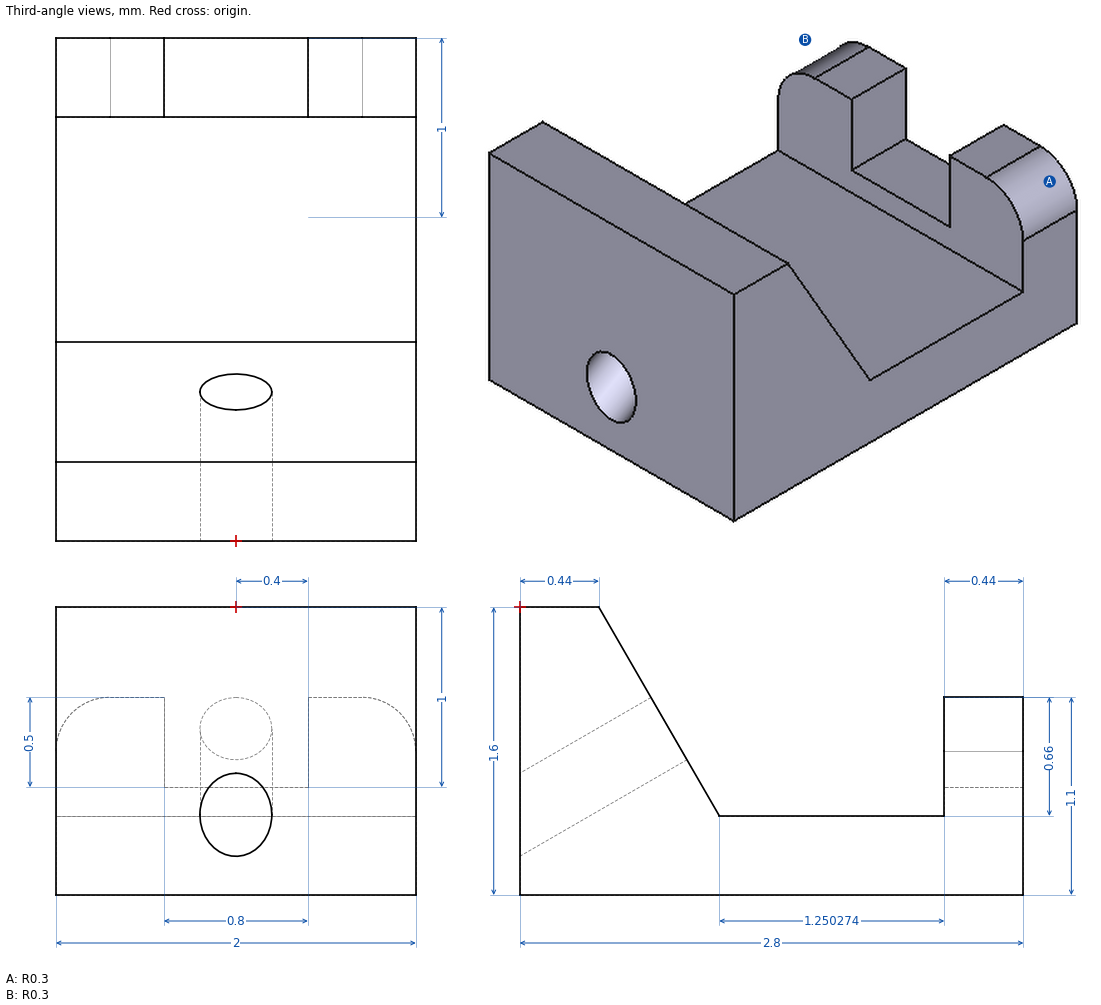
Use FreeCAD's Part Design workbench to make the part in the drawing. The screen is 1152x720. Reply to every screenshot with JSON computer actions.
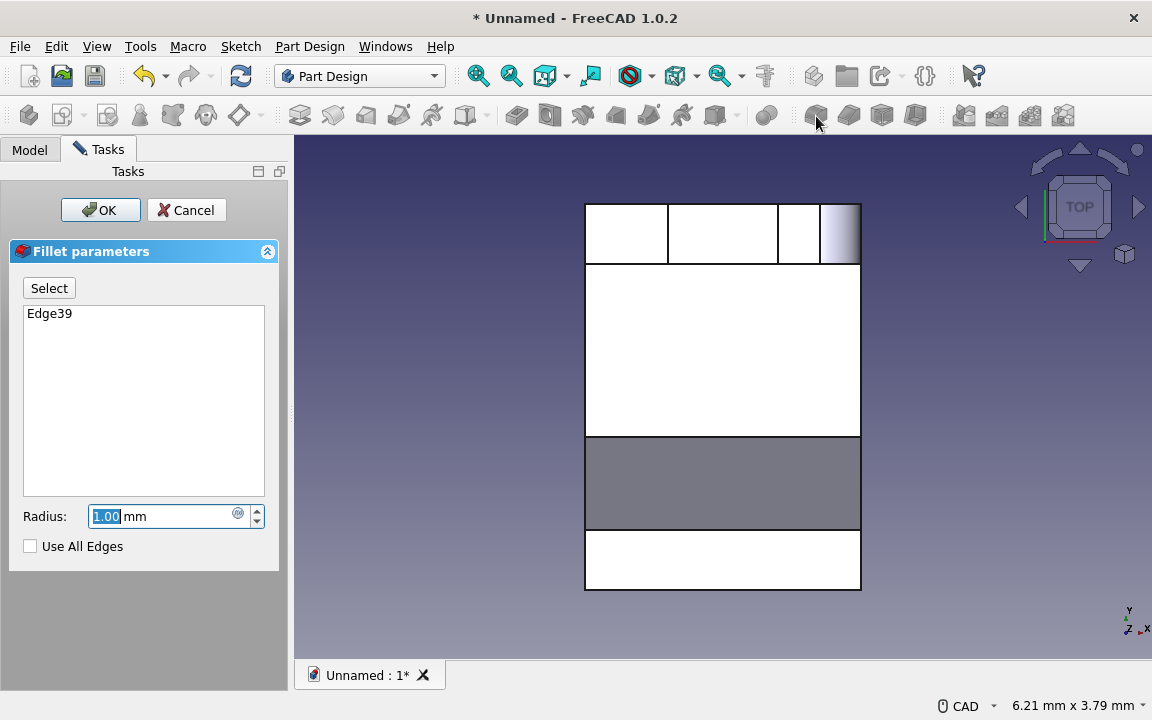
{"action": "type", "text": "0.3"}
{"action": "key", "text": "Tab"}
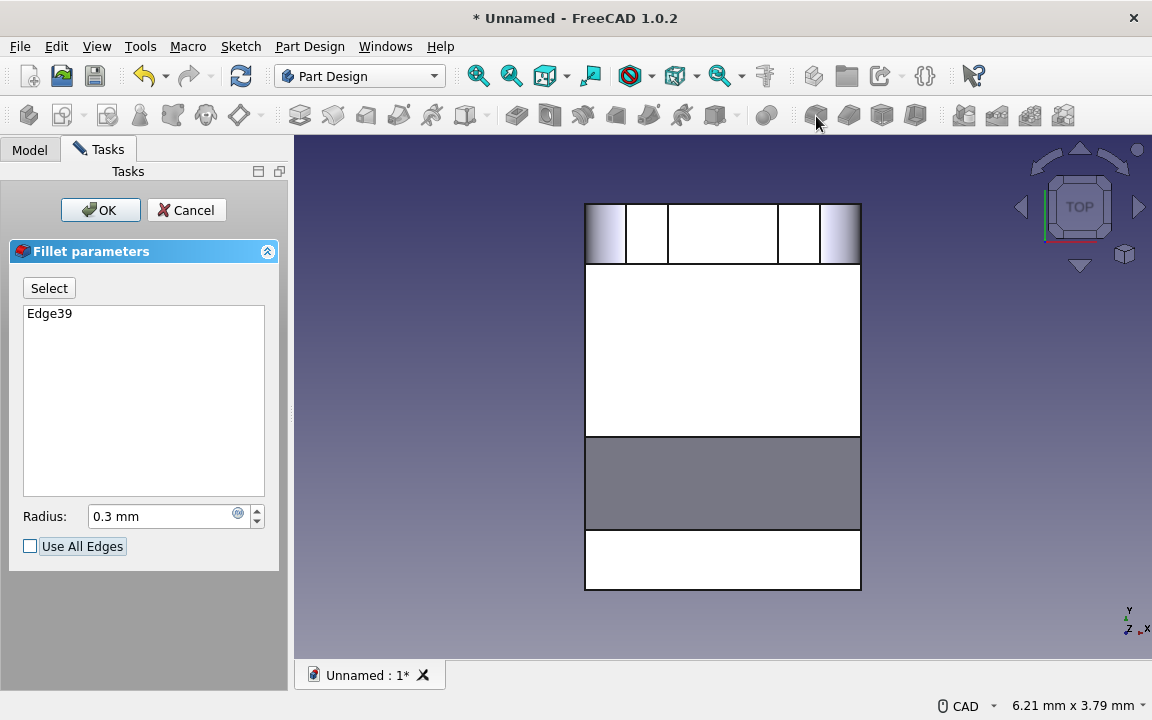
{"action": "left_click", "coordinate": [101, 210]}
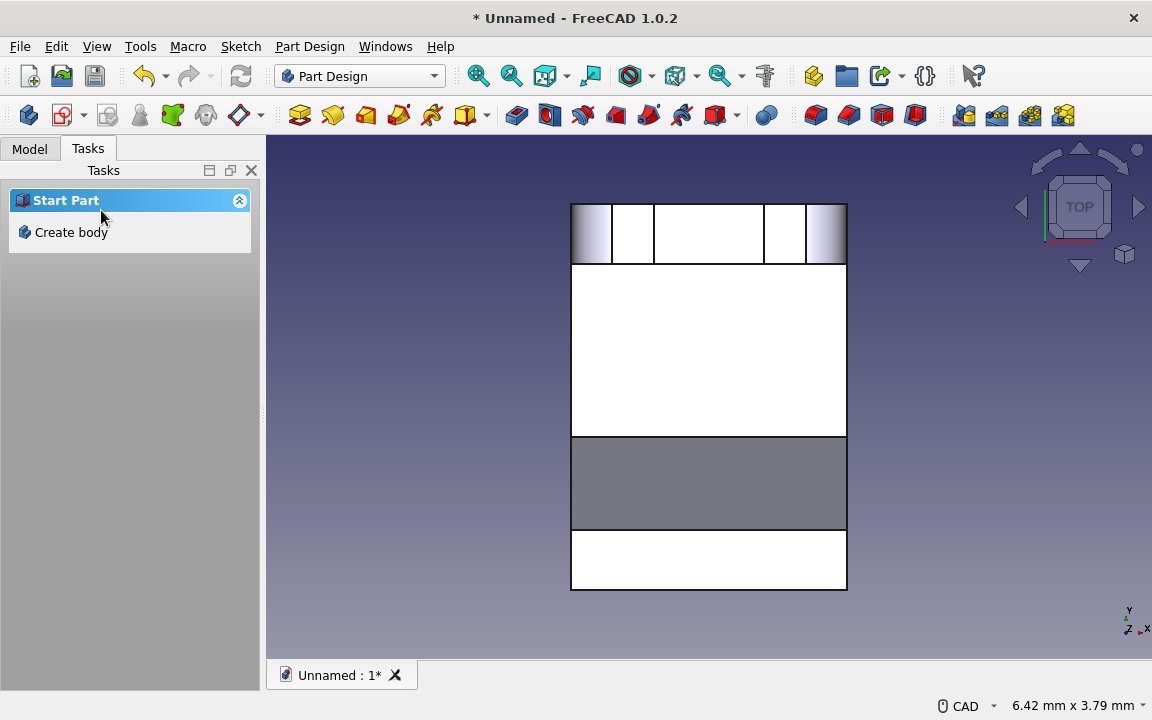
{"action": "left_click", "coordinate": [670, 482]}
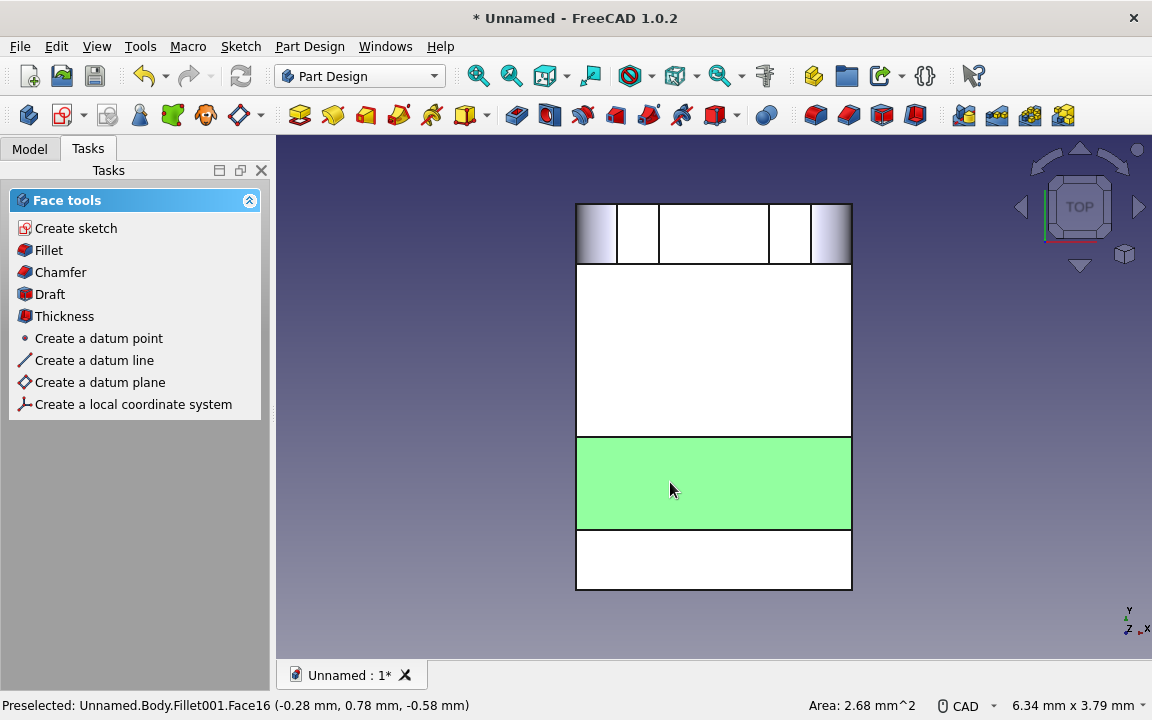
{"action": "left_click", "coordinate": [62, 116]}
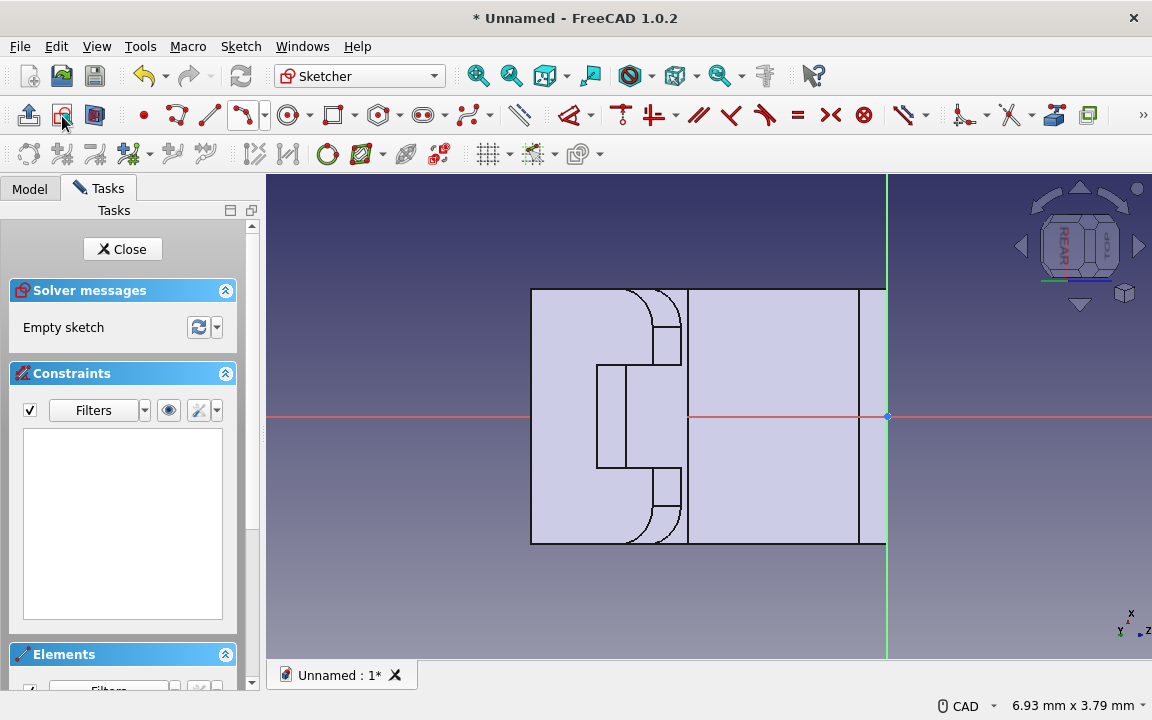
{"action": "scroll", "coordinate": [783, 416], "scroll_direction": "up", "scroll_amount": 9}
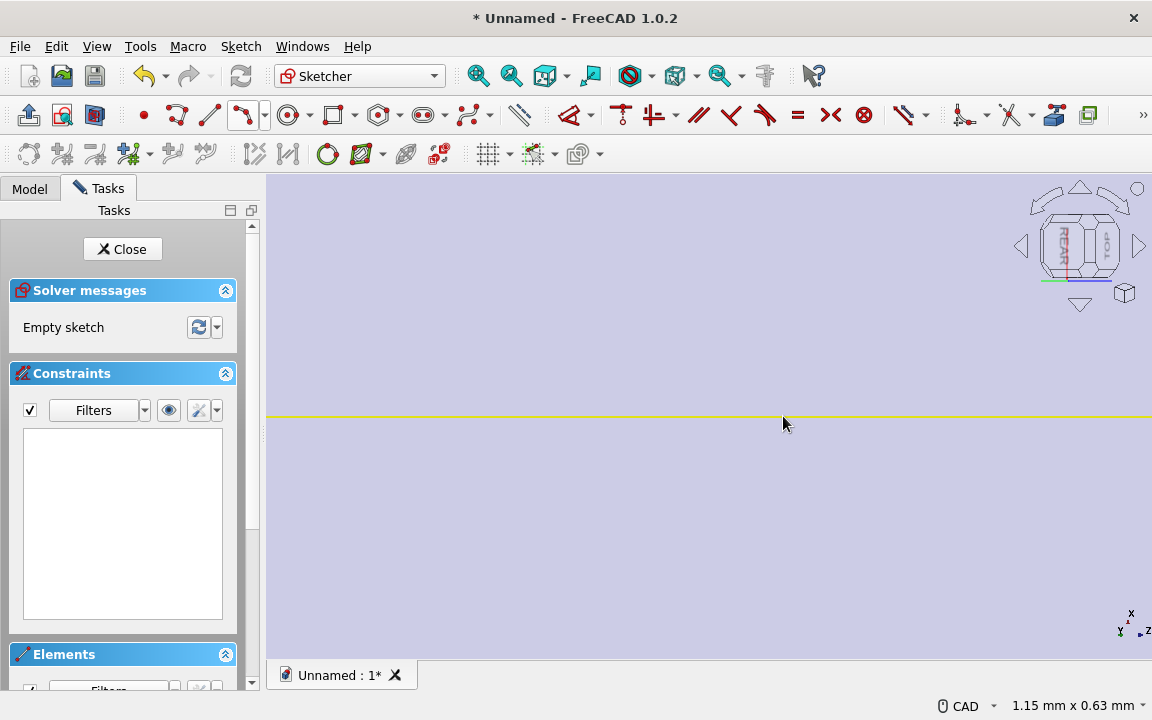
{"action": "key", "text": "g c"}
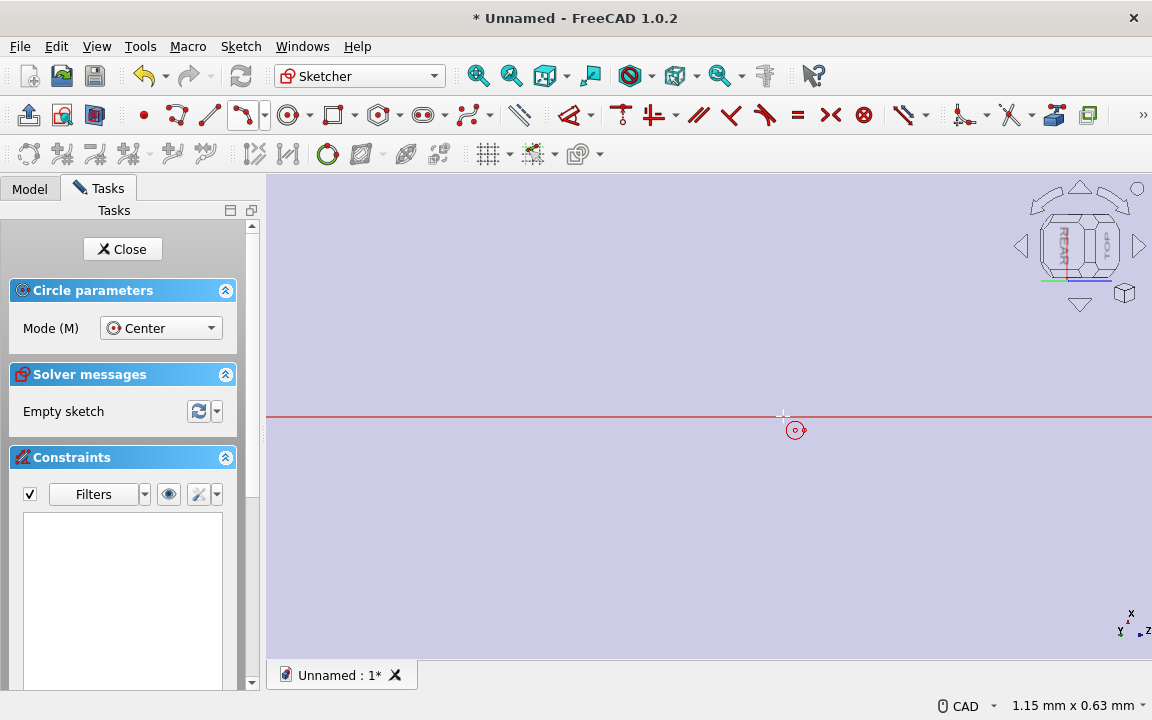
{"action": "left_click", "coordinate": [637, 416]}
{"action": "left_click", "coordinate": [746, 307]}
{"action": "key", "text": "Escape"}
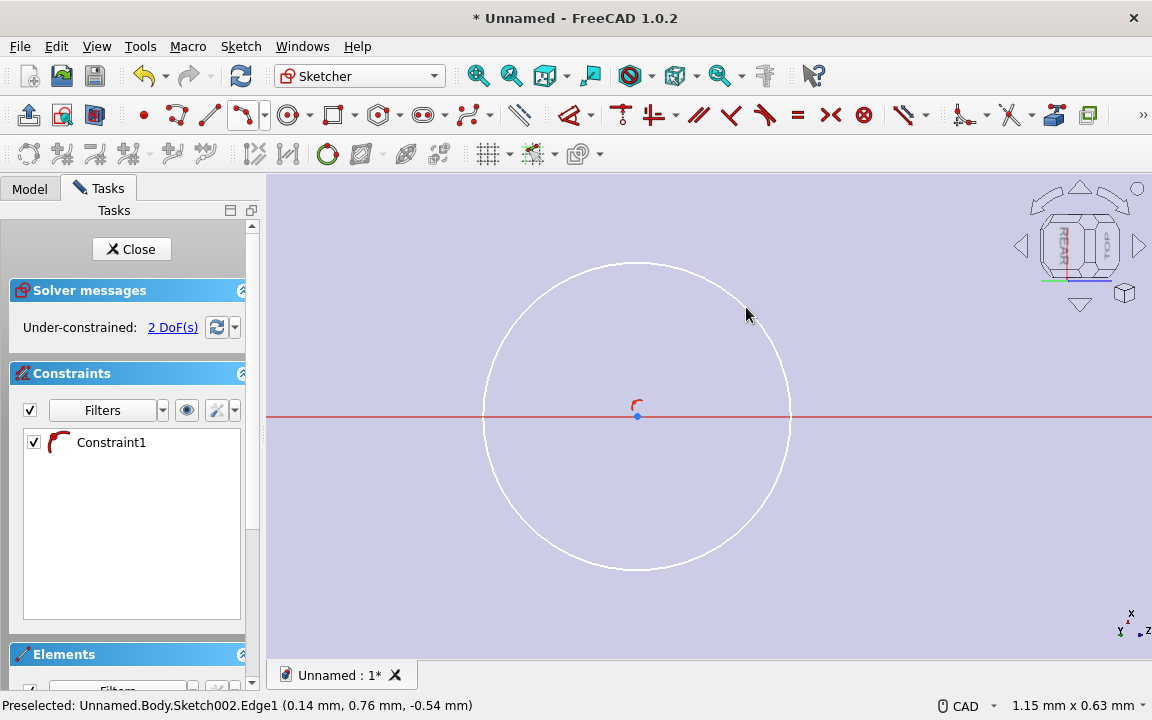
{"action": "key", "text": "d"}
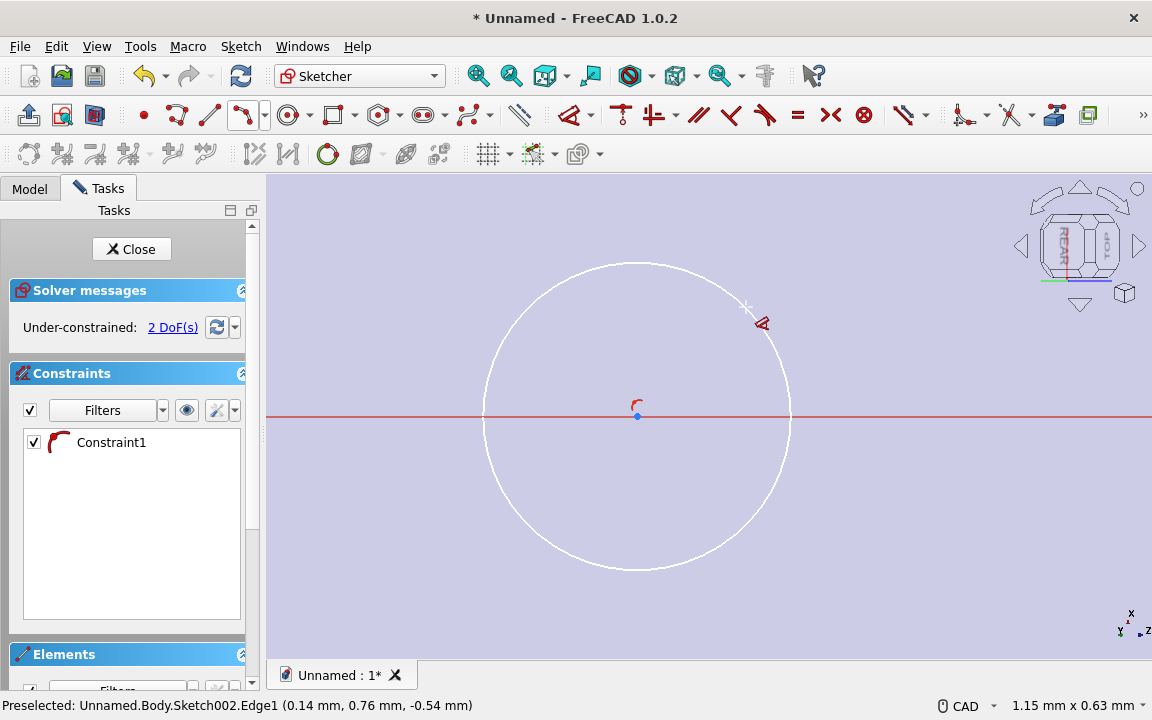
{"action": "left_click", "coordinate": [745, 307]}
{"action": "left_click", "coordinate": [767, 284]}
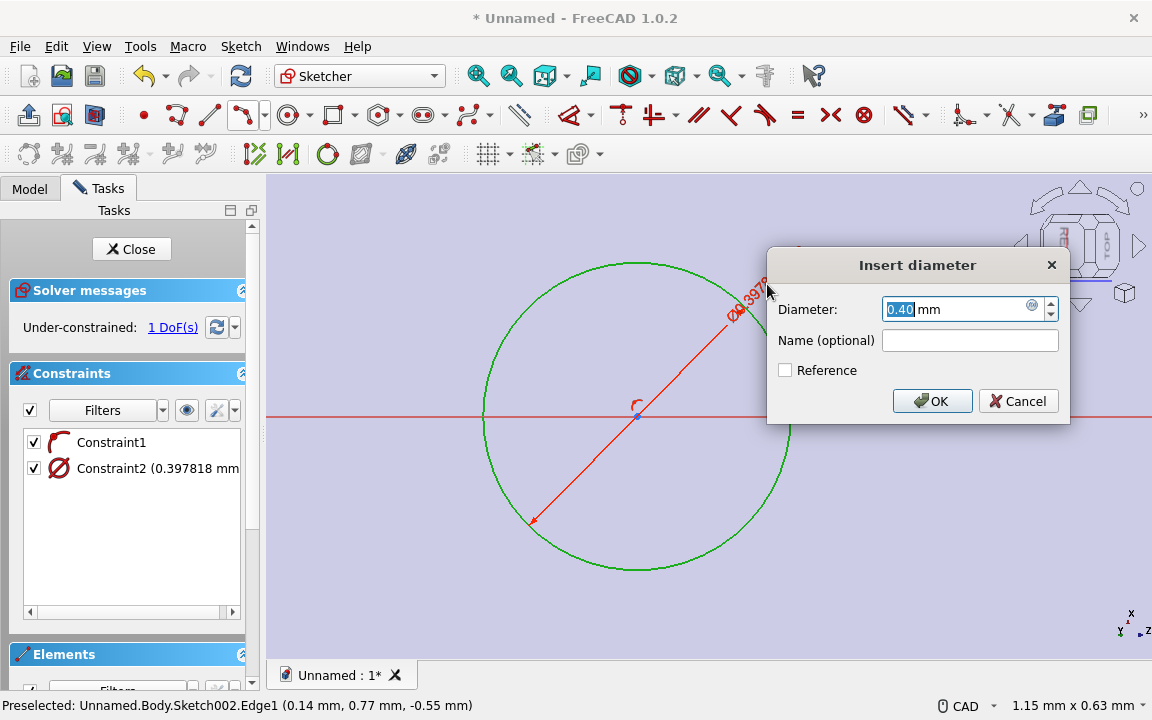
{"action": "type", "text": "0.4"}
{"action": "key", "text": "Return"}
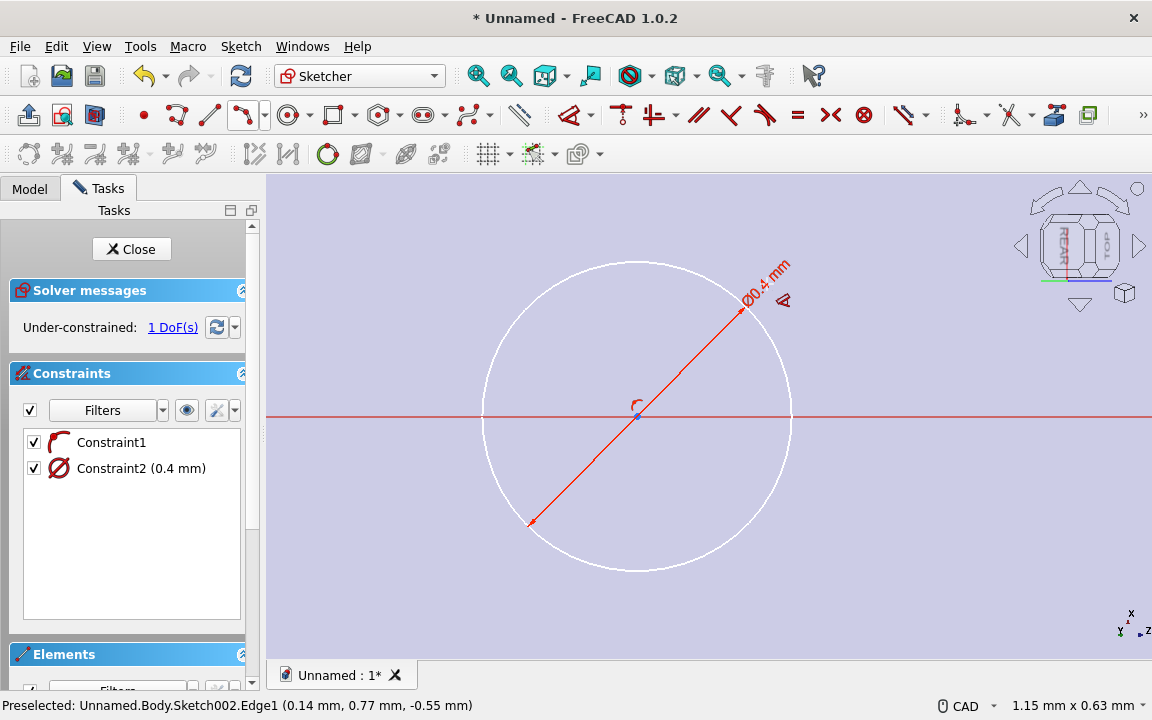
{"action": "left_click", "coordinate": [637, 416]}
{"action": "left_click", "coordinate": [812, 450]}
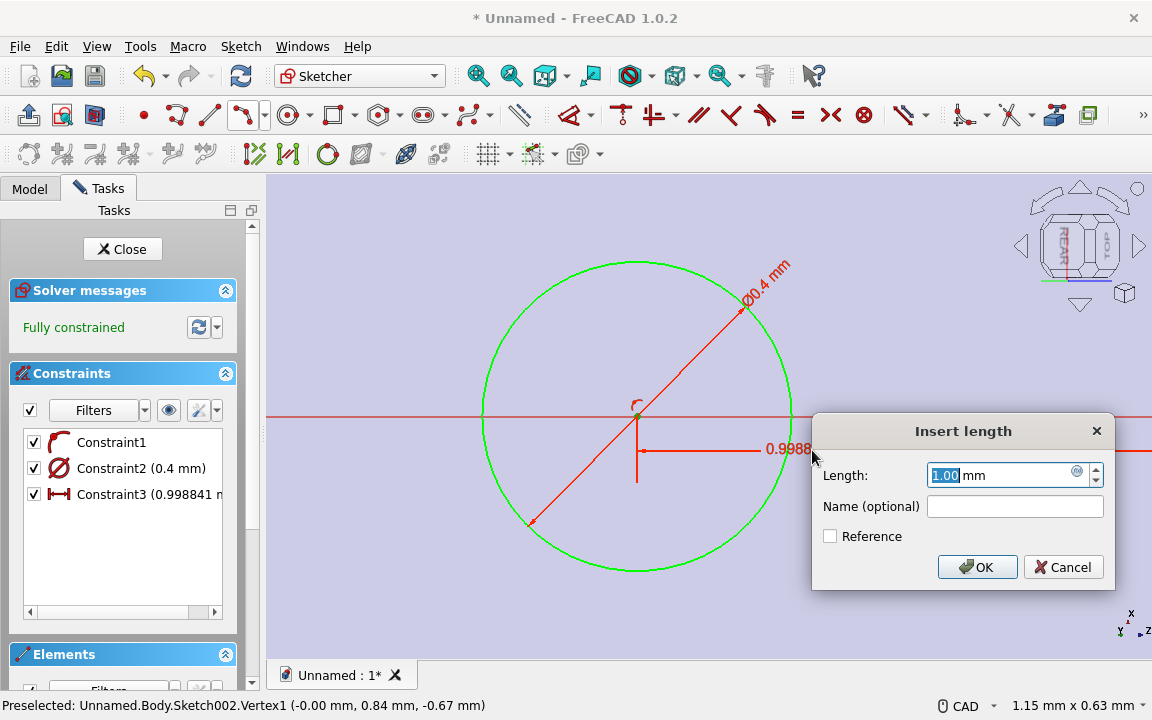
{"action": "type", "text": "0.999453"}
{"action": "key", "text": "Return"}
{"action": "key", "text": "Escape"}